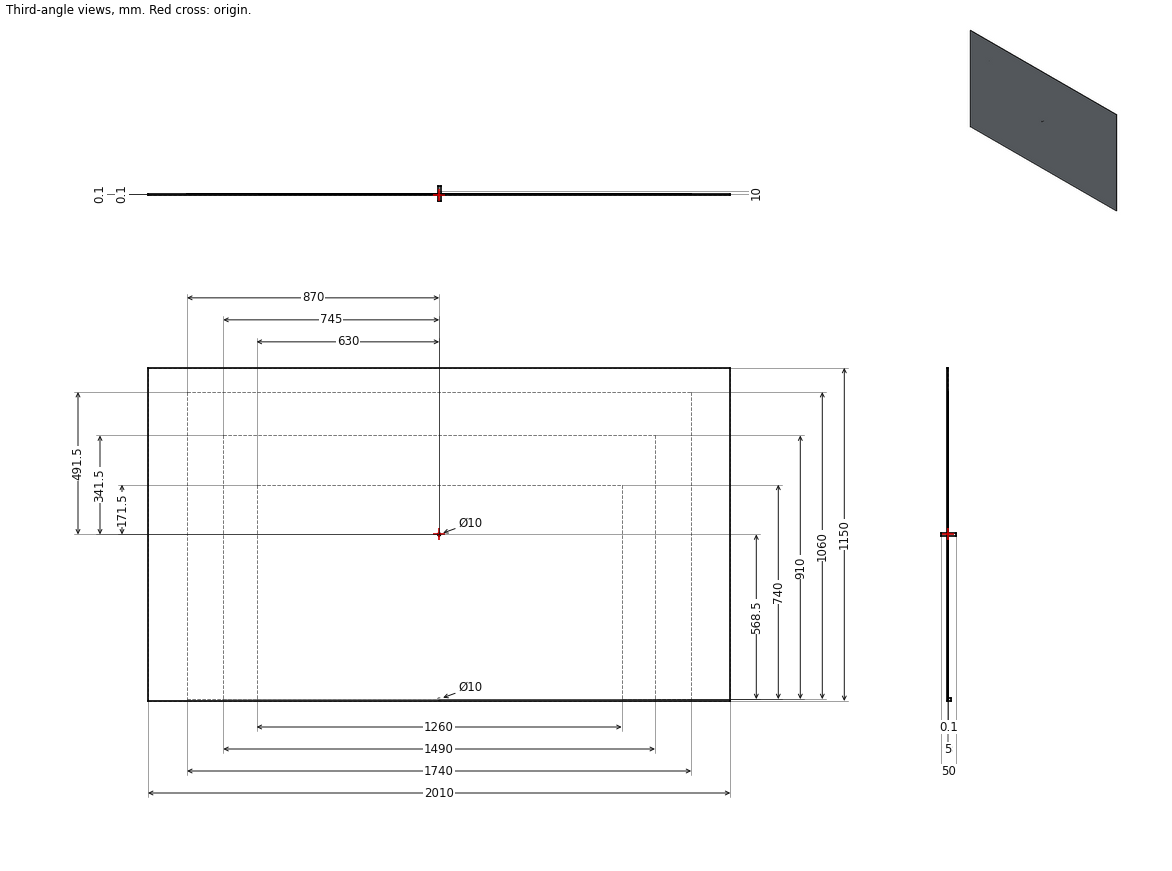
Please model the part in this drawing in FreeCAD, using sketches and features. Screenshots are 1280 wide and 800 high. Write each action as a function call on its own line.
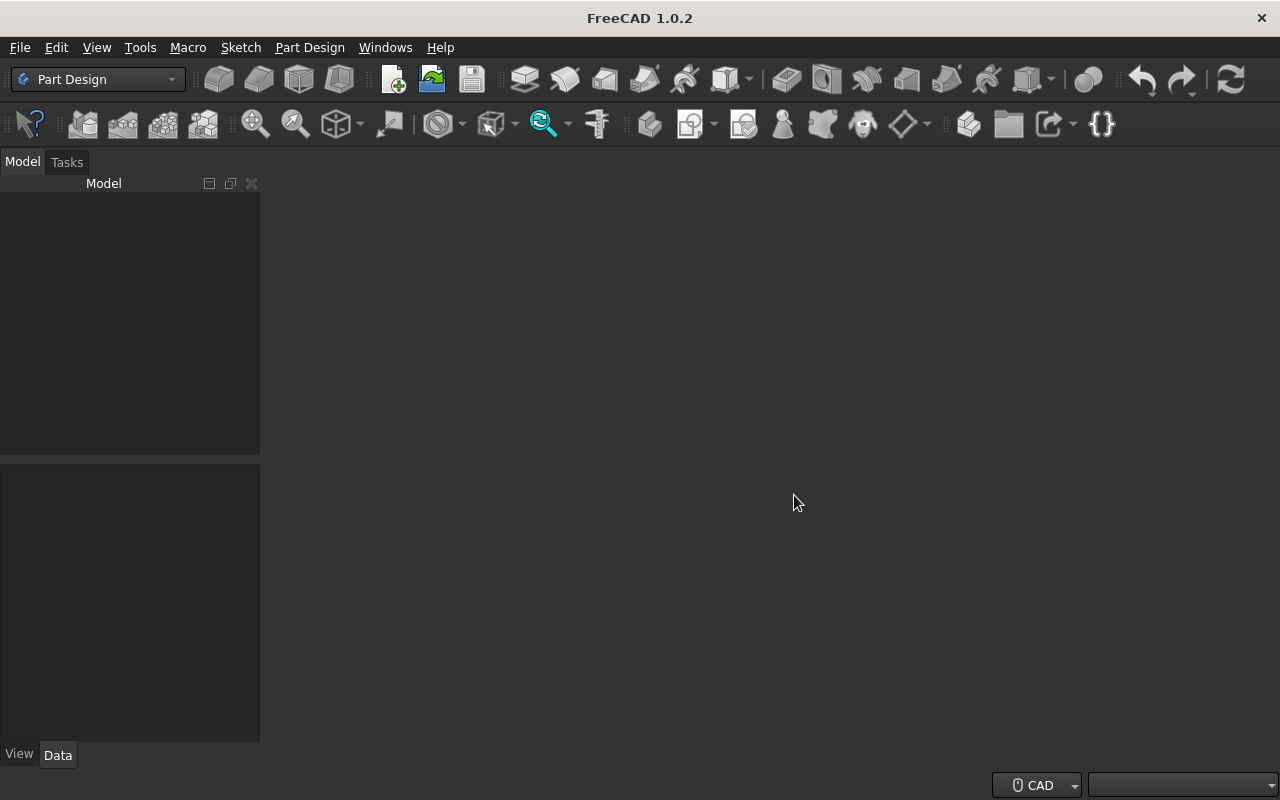
click(392, 80)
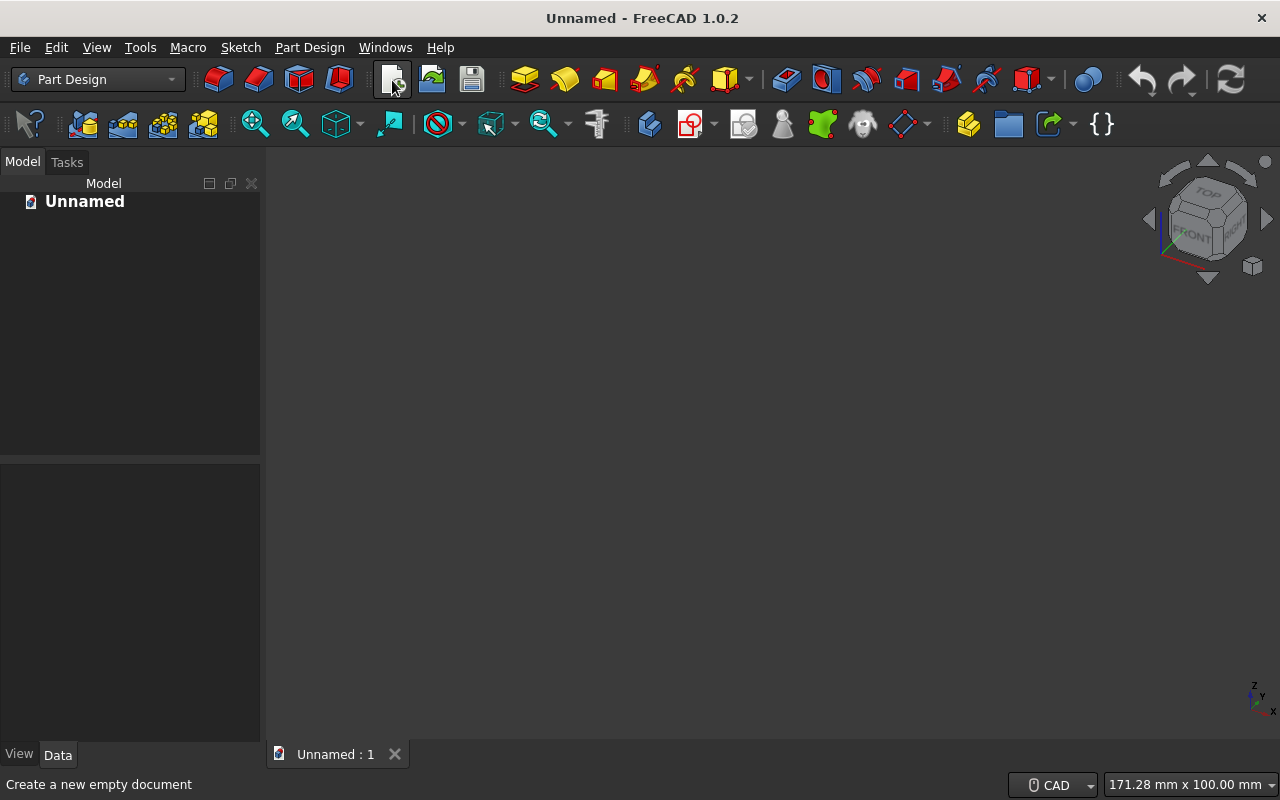
click(690, 124)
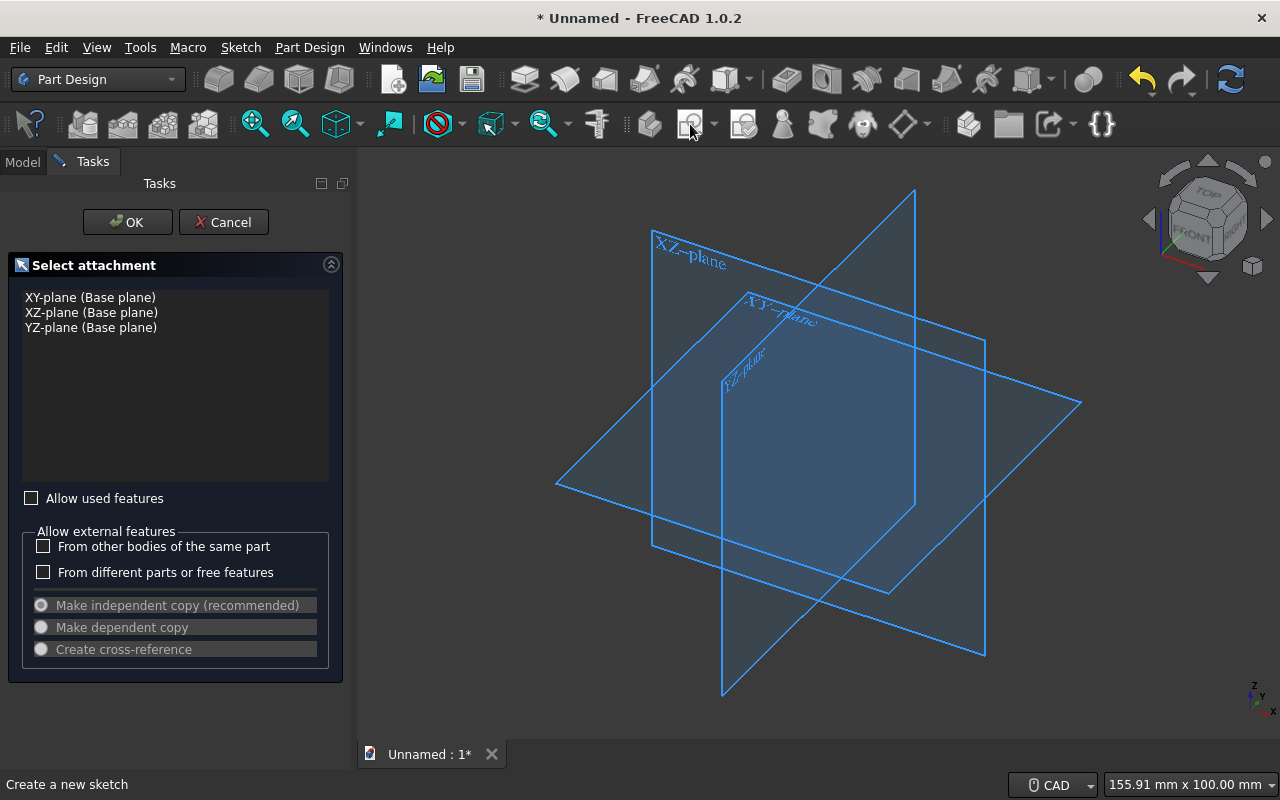
click(82, 312)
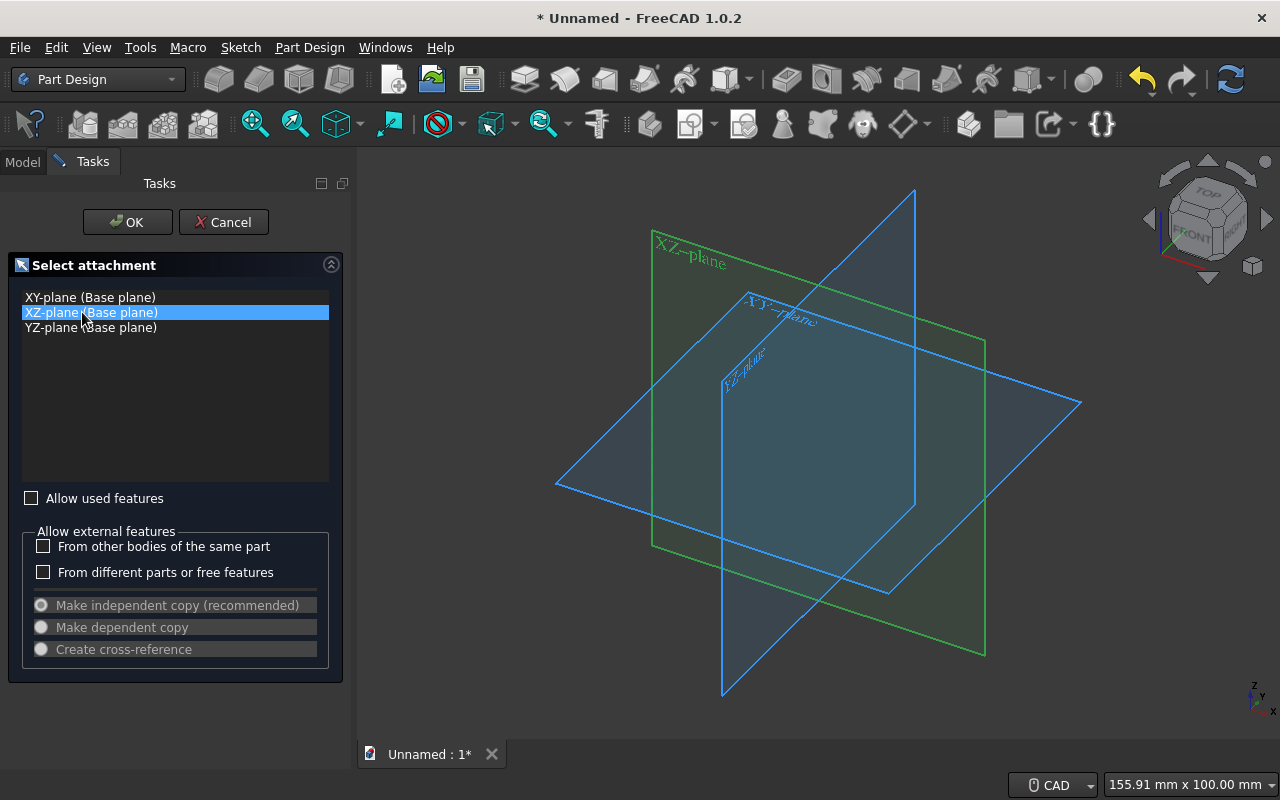
click(128, 222)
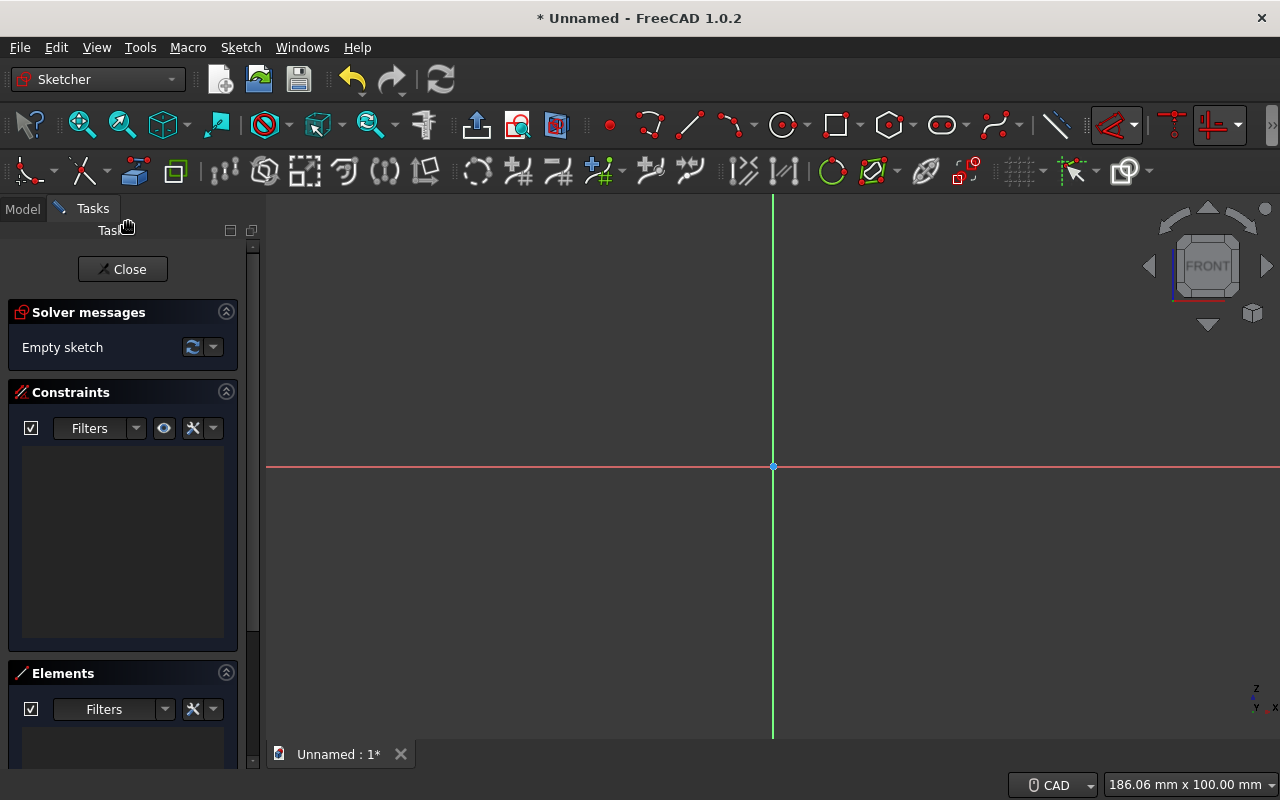
scroll(701, 466, down, 15)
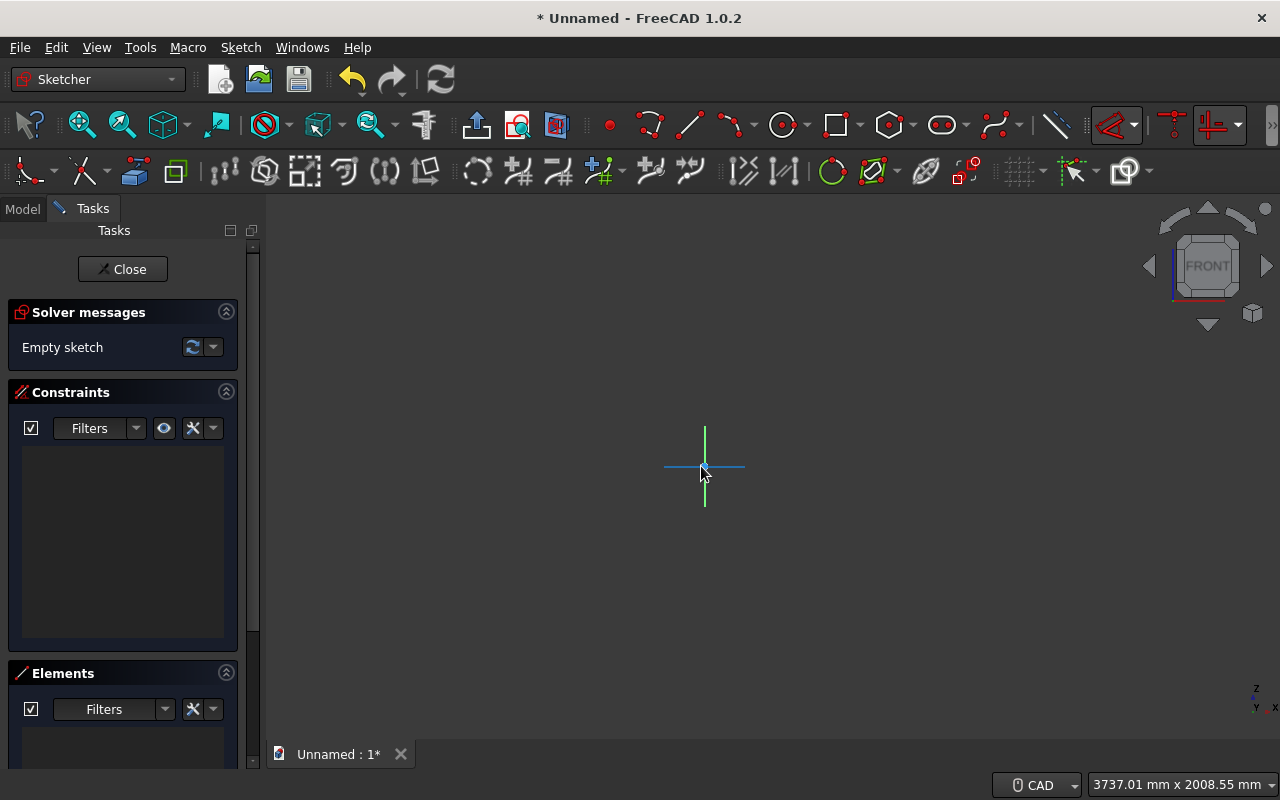
click(862, 126)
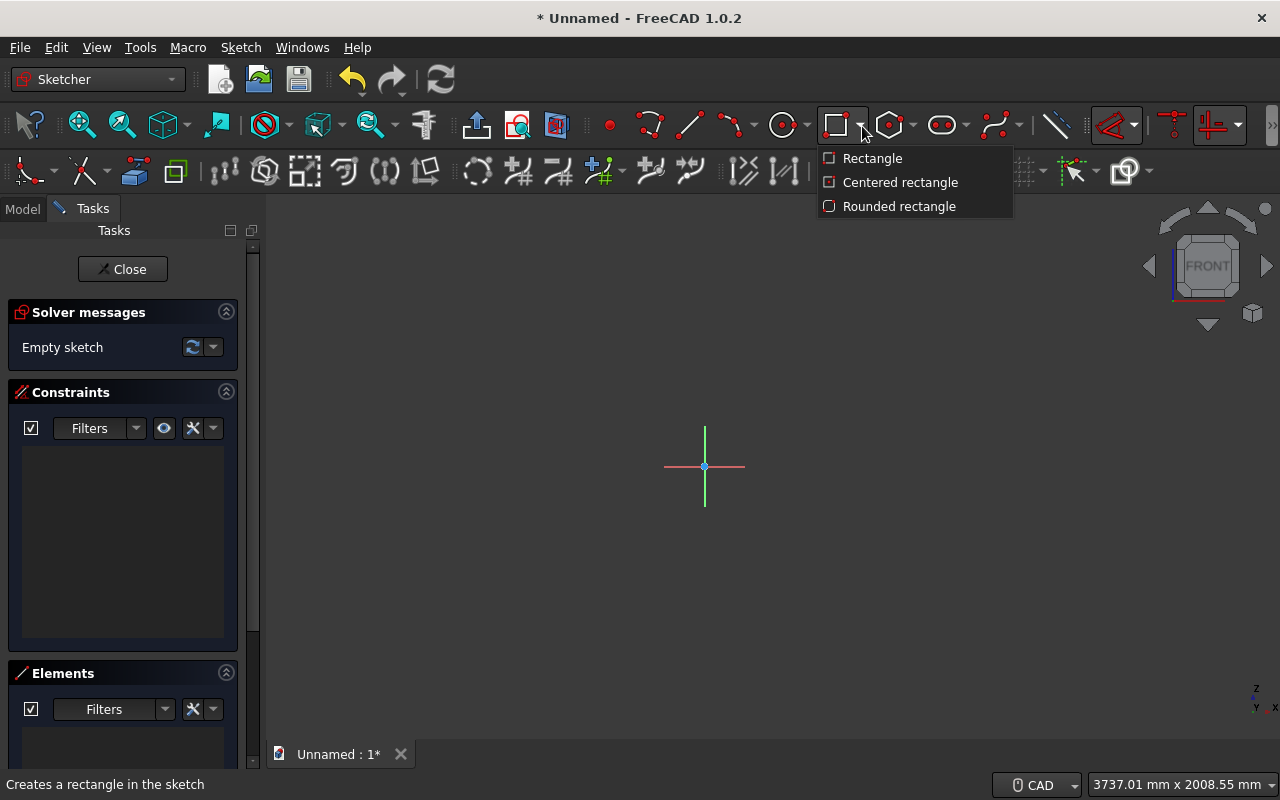
click(916, 182)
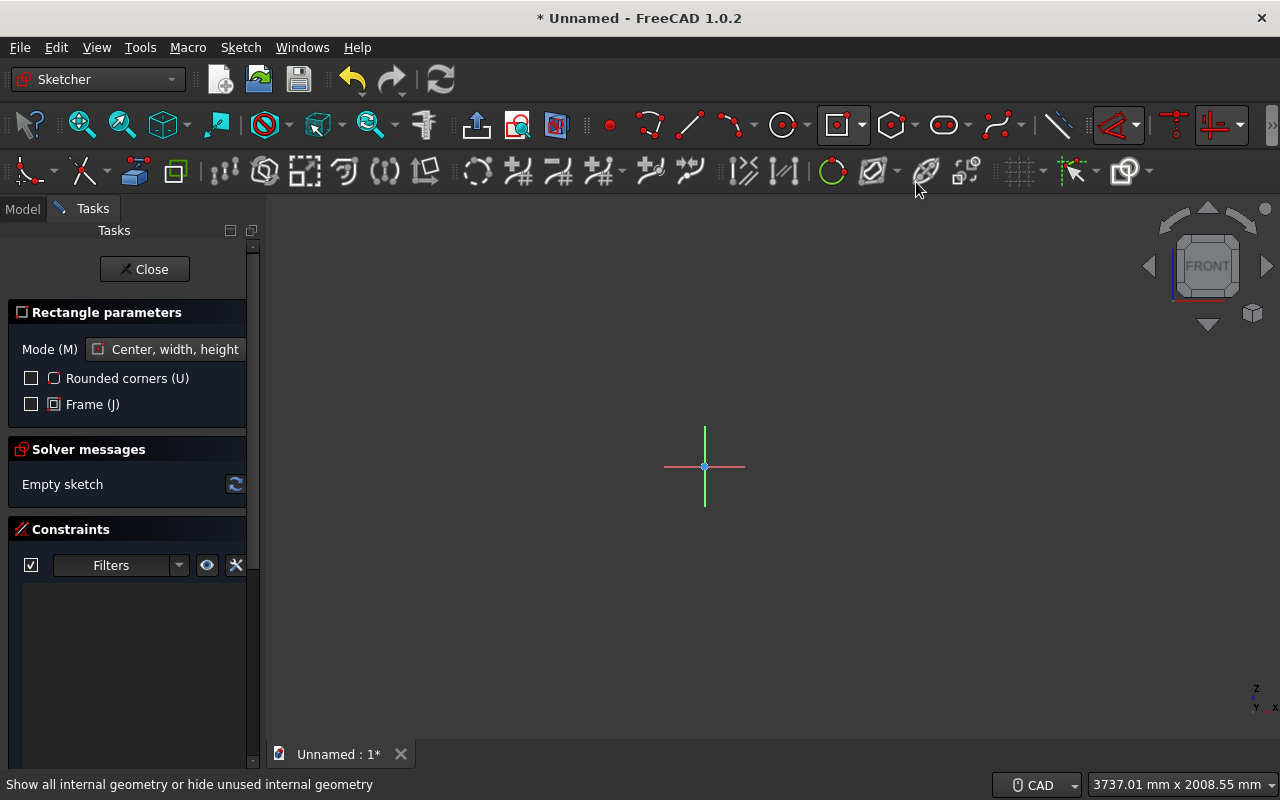
click(705, 466)
move(978, 310)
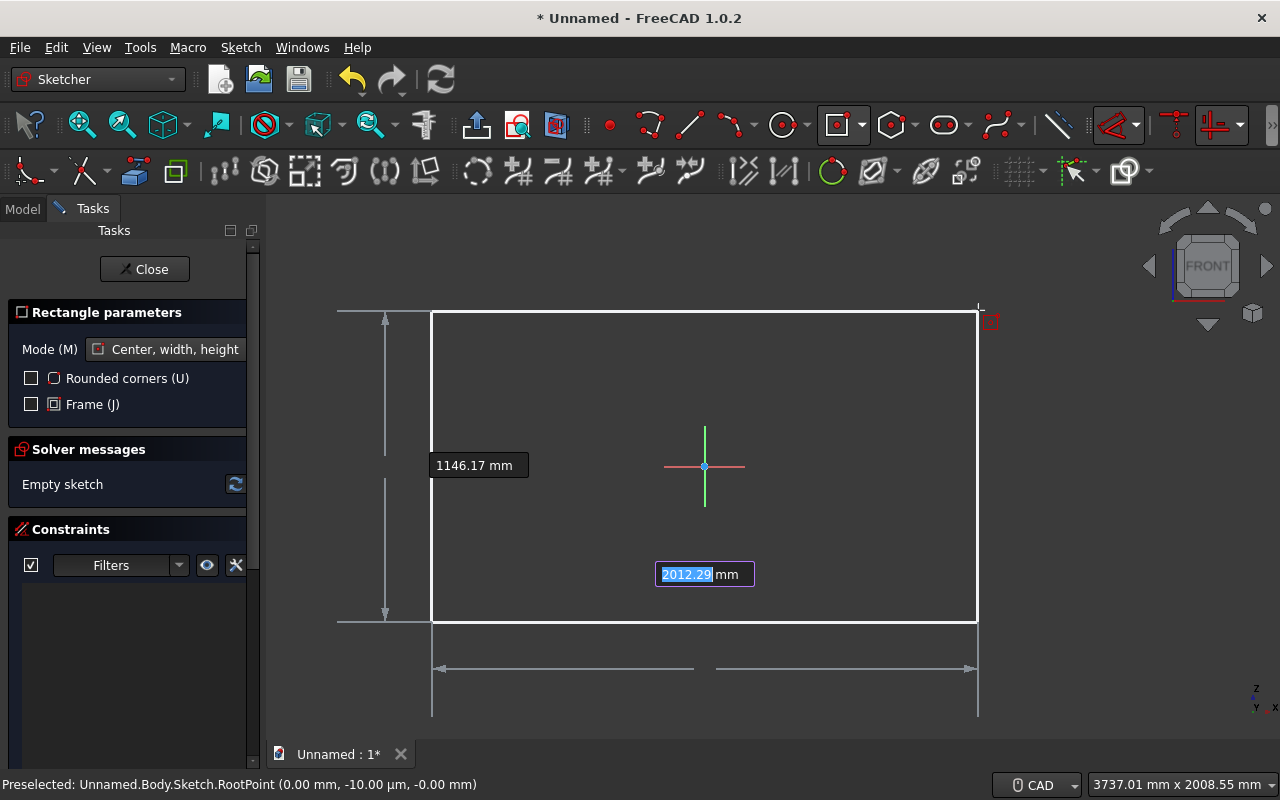
text(2010)
key(Tab)
text(1150)
key(Return)
key(Escape)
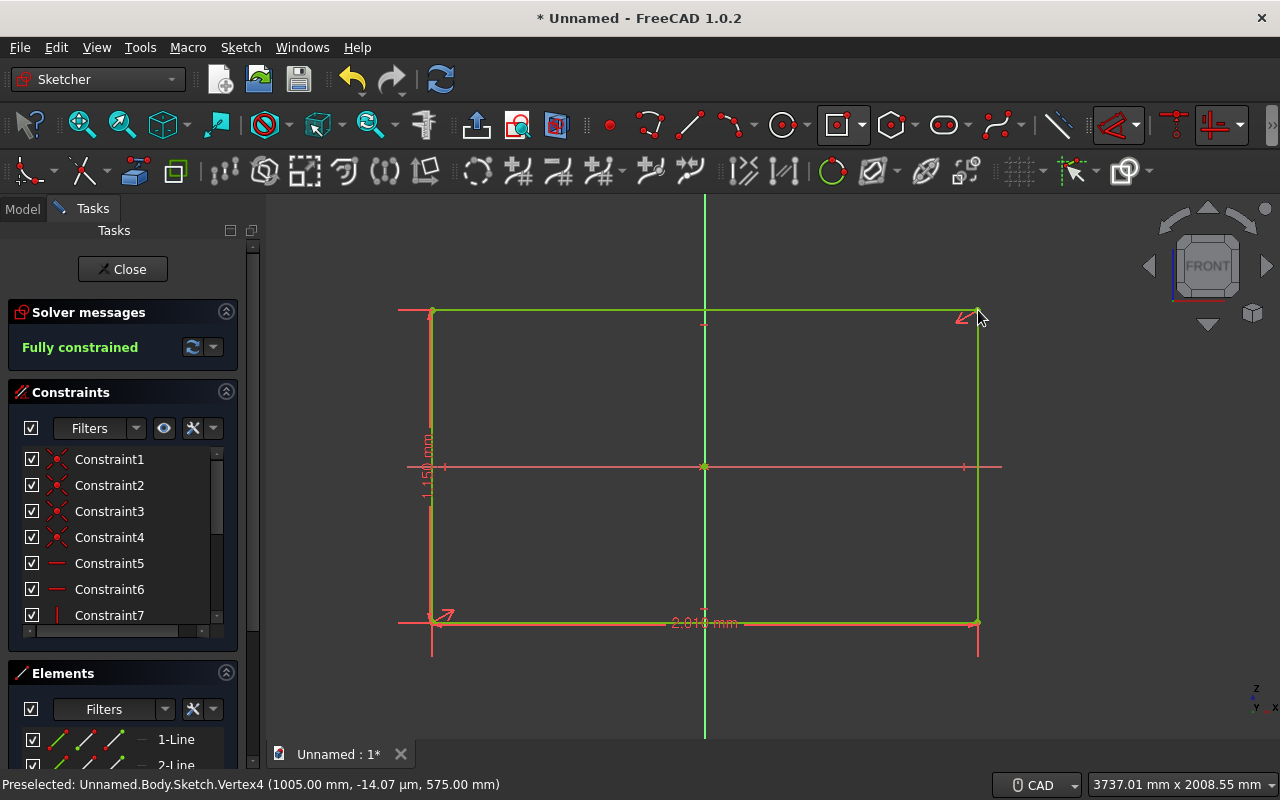
click(123, 269)